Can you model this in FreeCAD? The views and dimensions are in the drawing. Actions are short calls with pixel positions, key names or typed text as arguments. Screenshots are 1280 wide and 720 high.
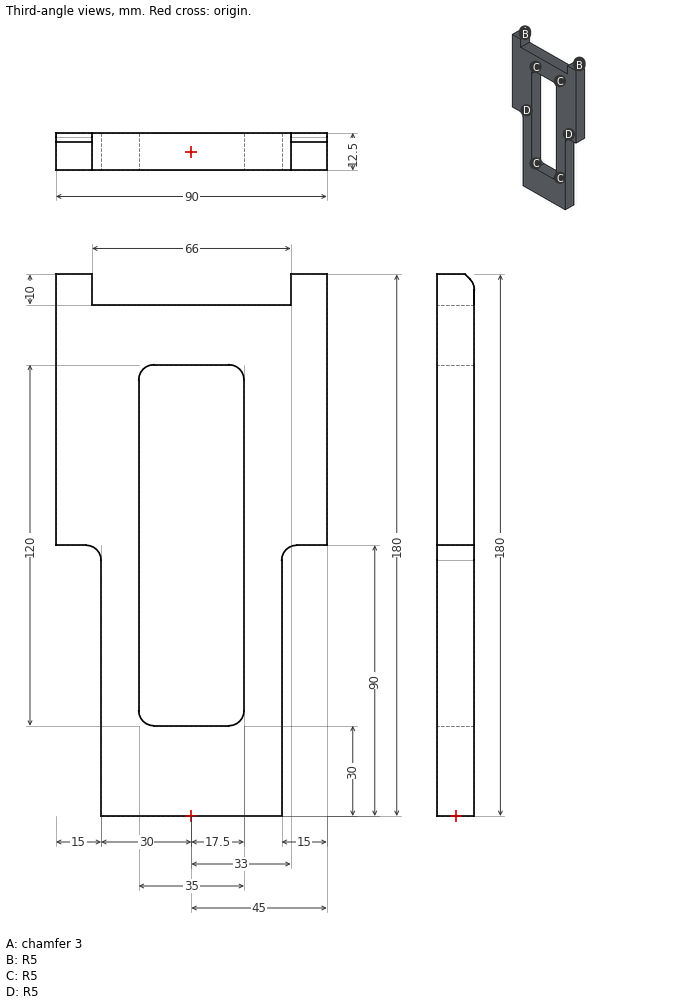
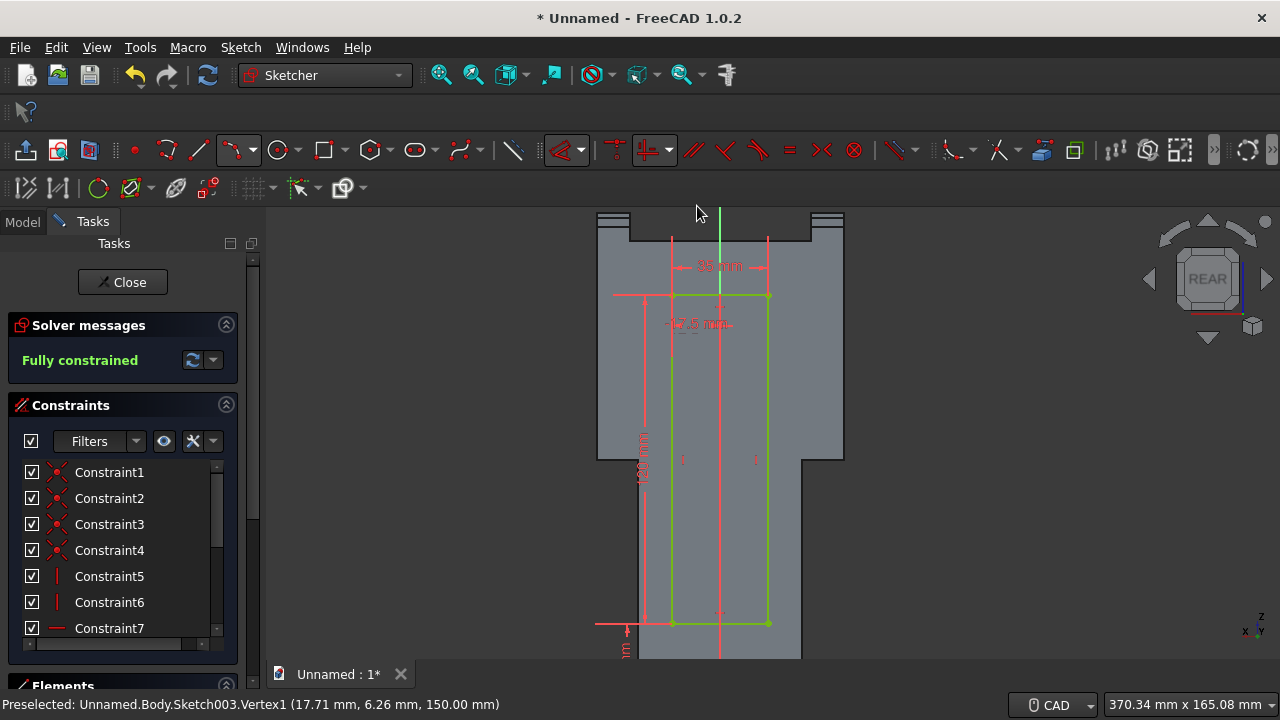
click(123, 282)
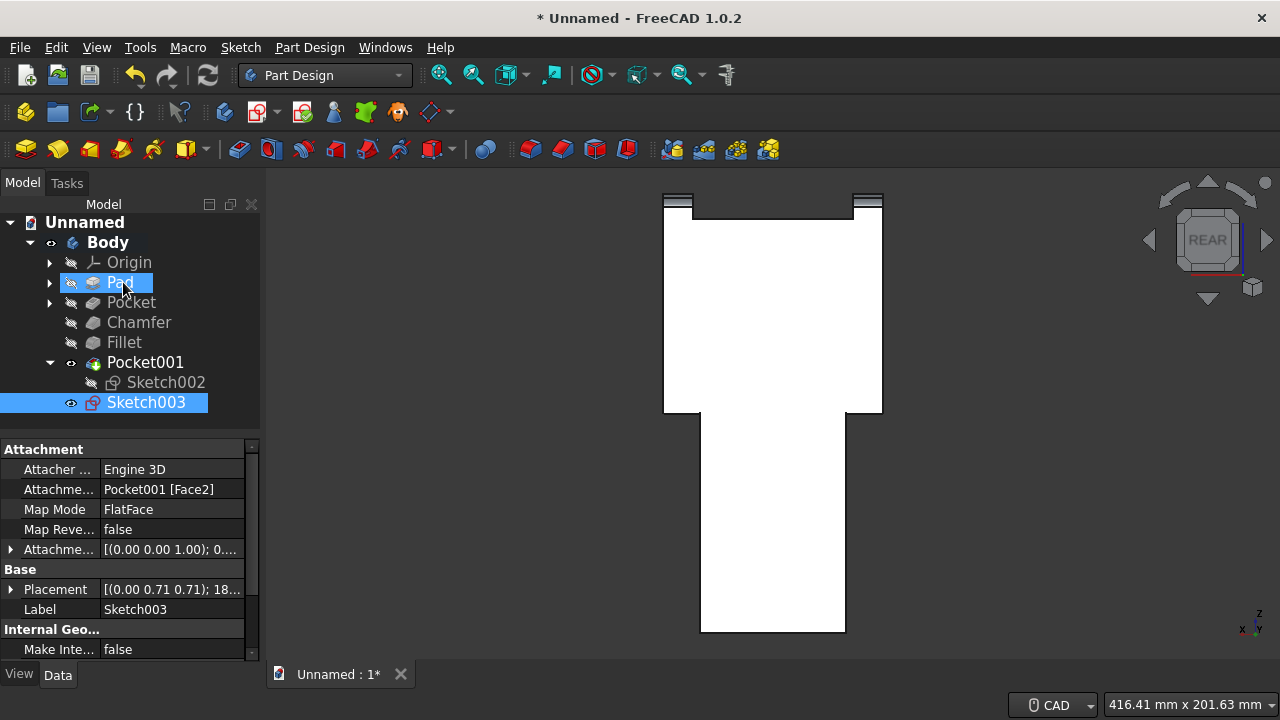
click(240, 150)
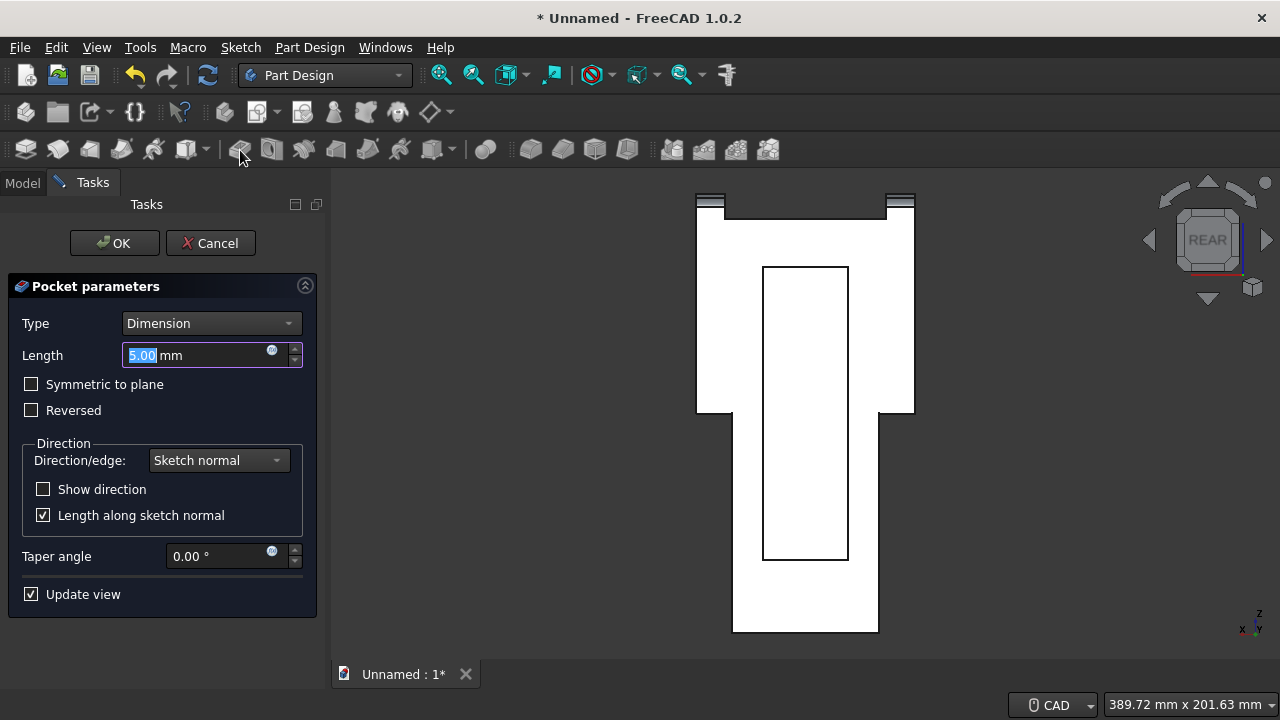
click(212, 324)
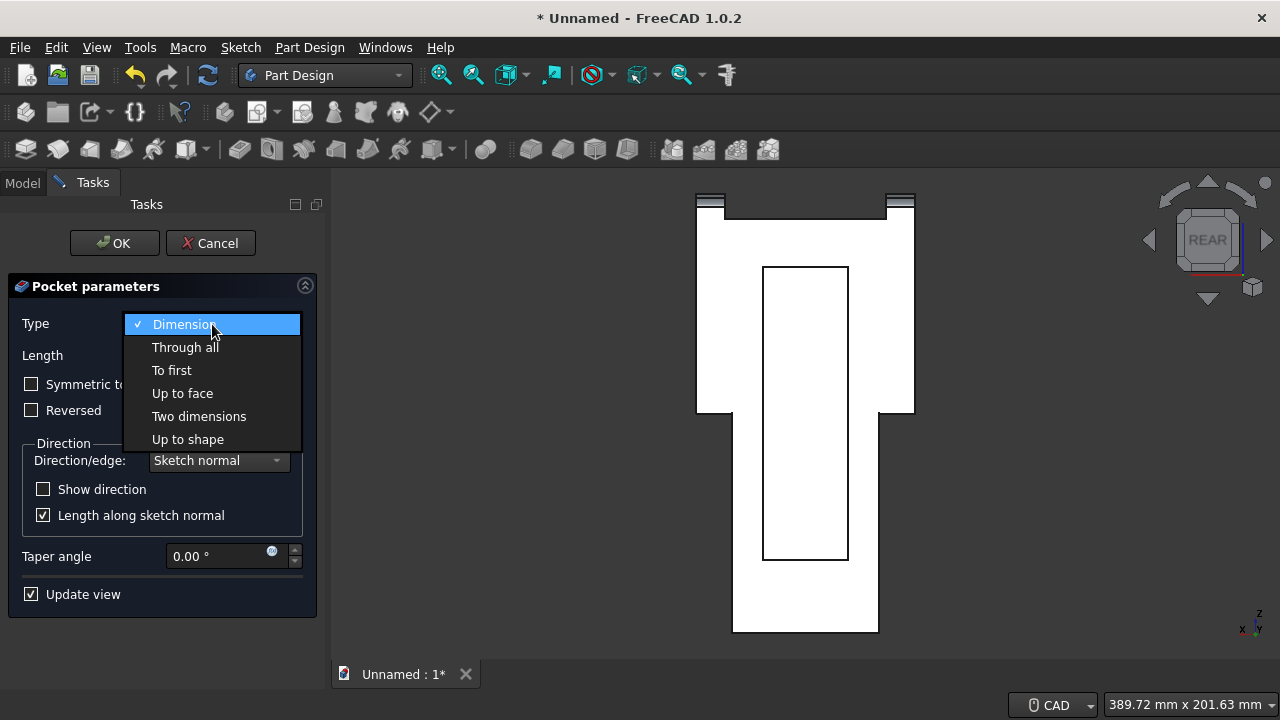
click(212, 348)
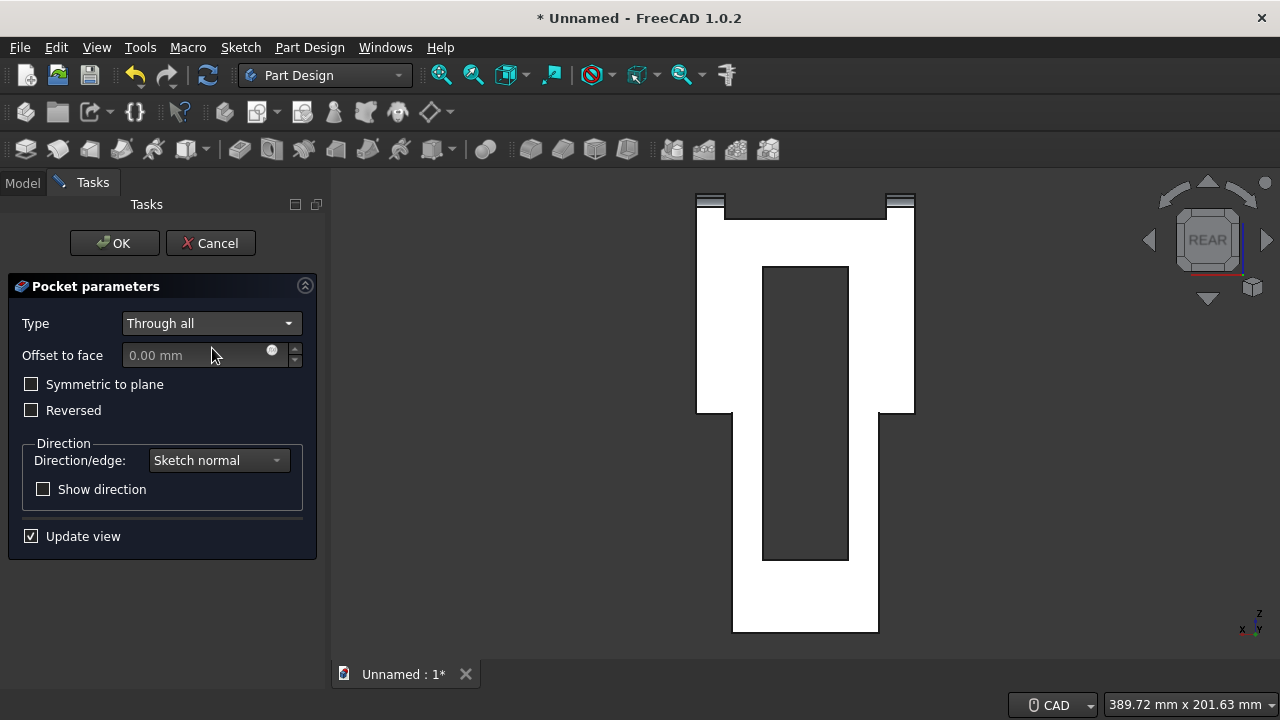
click(115, 243)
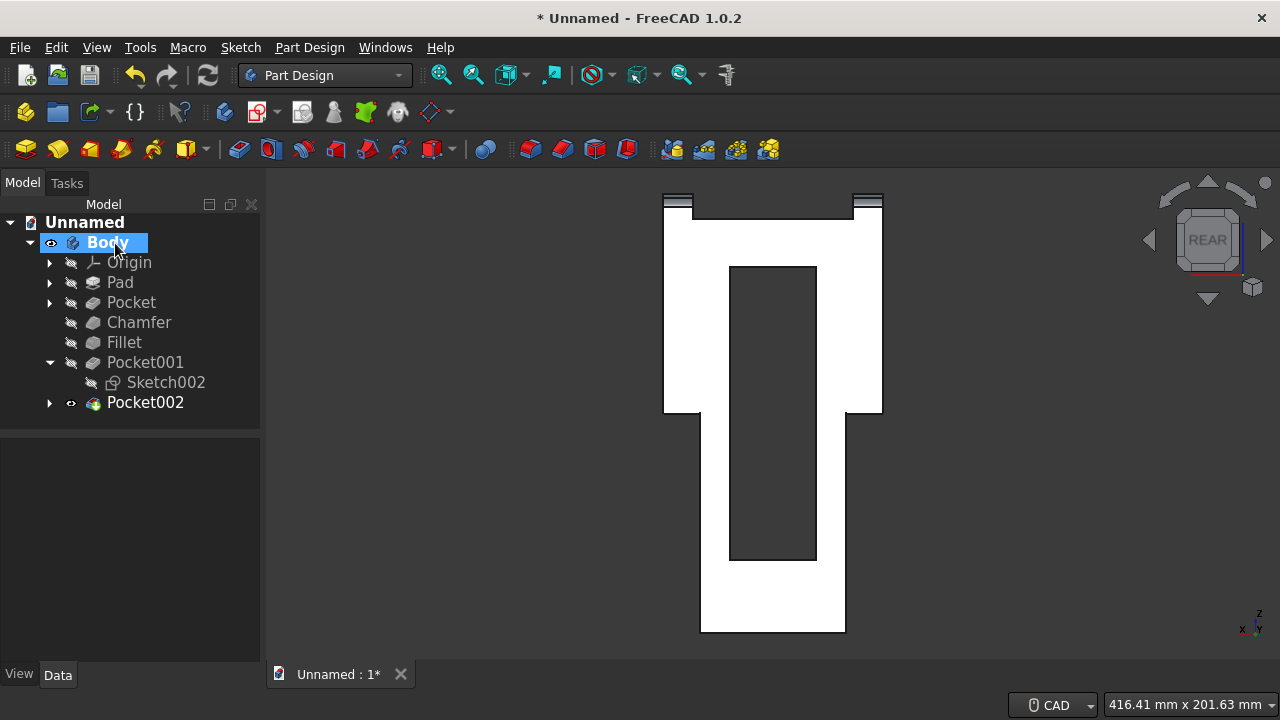
key(0)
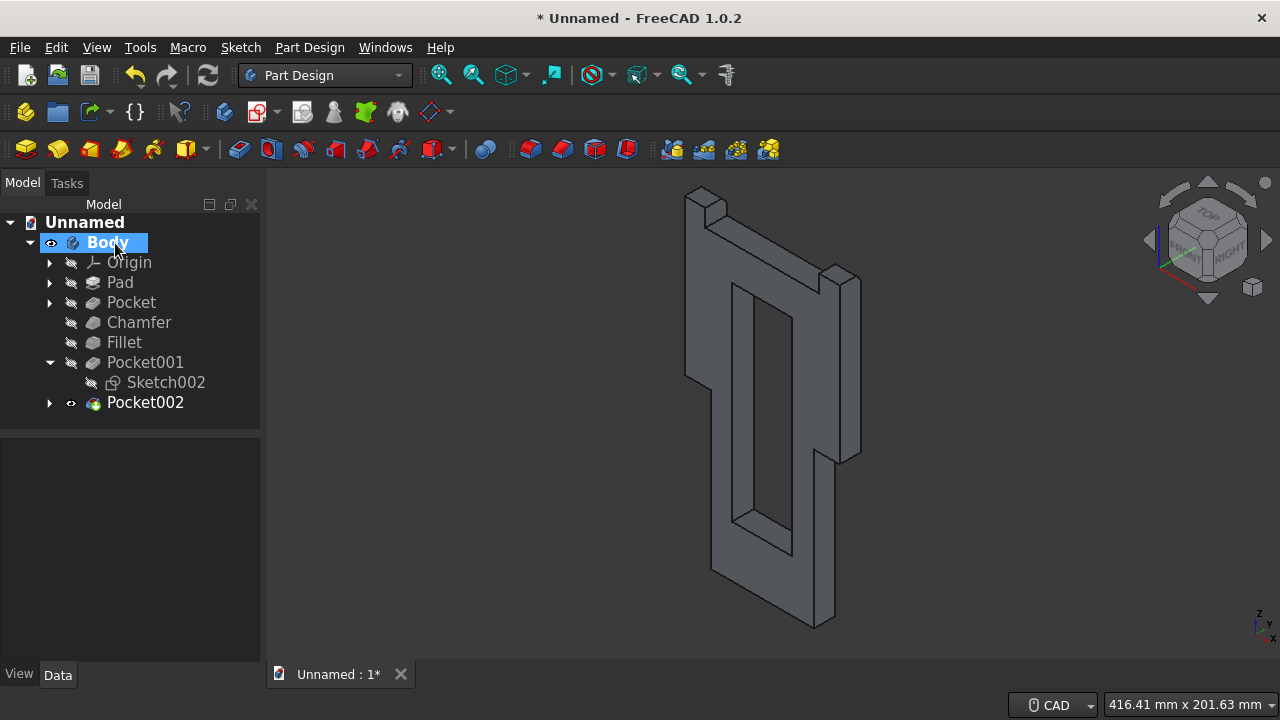
key(2)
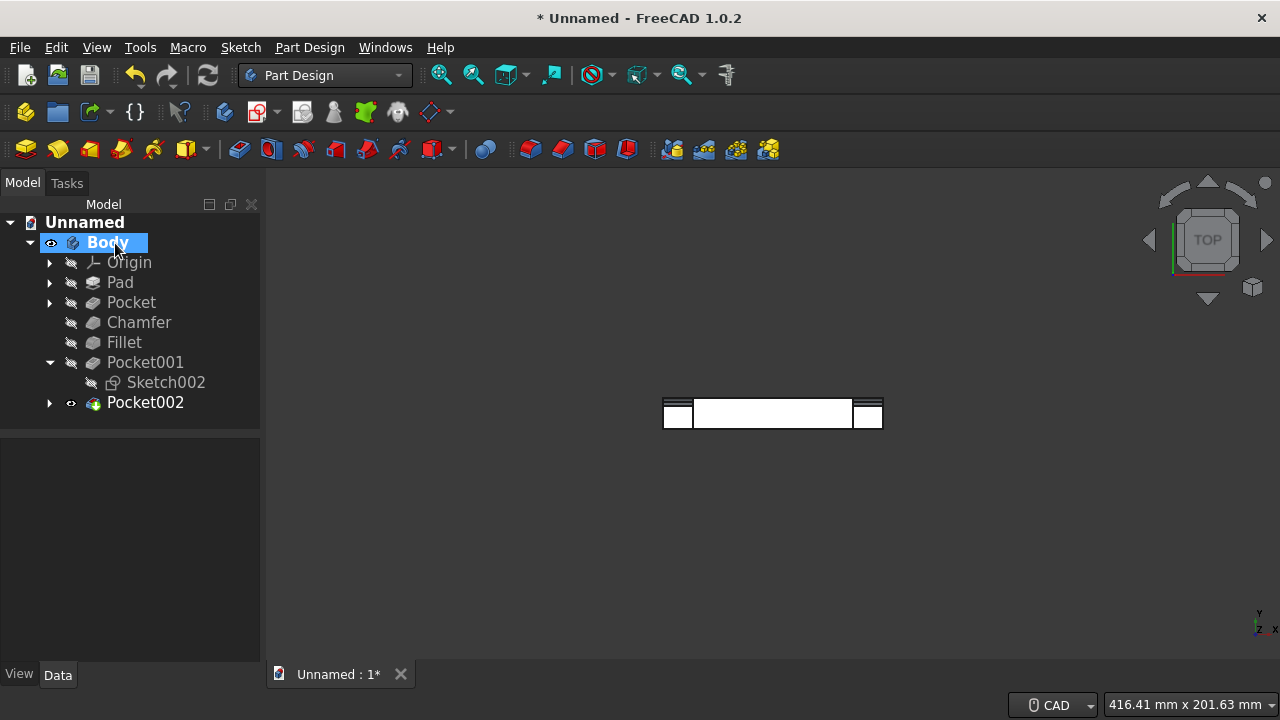
click(442, 76)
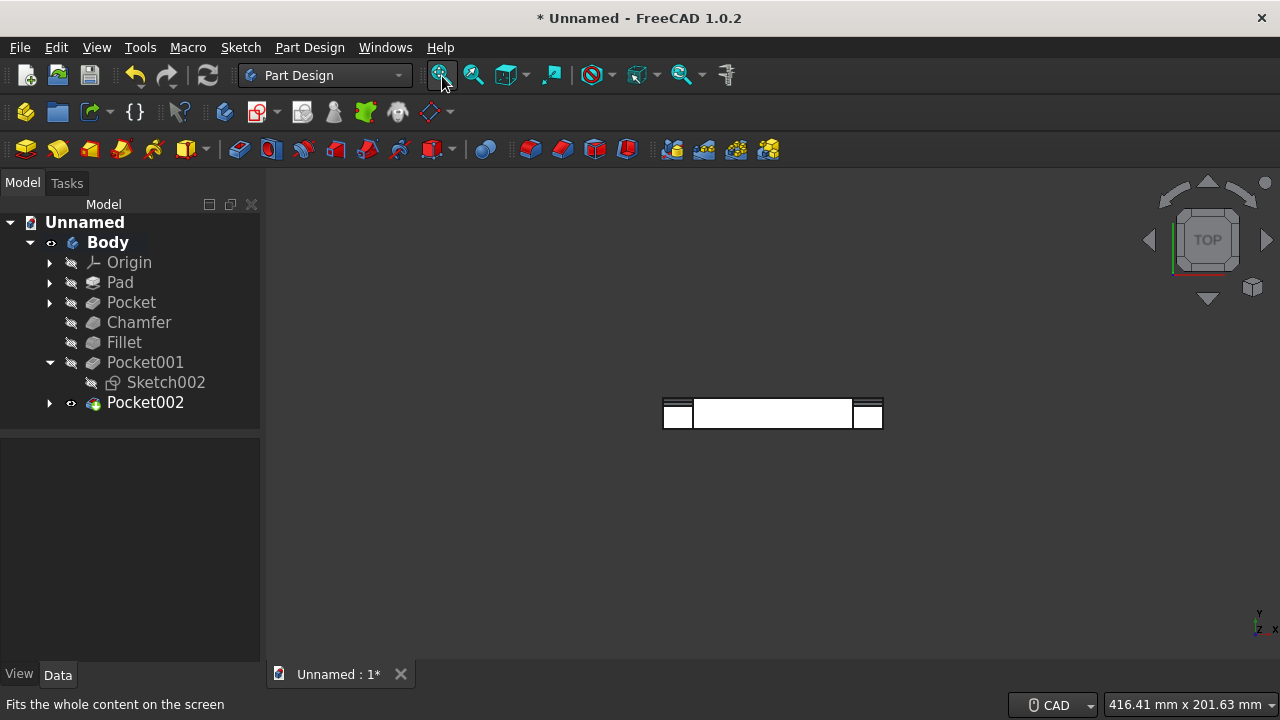
key(1)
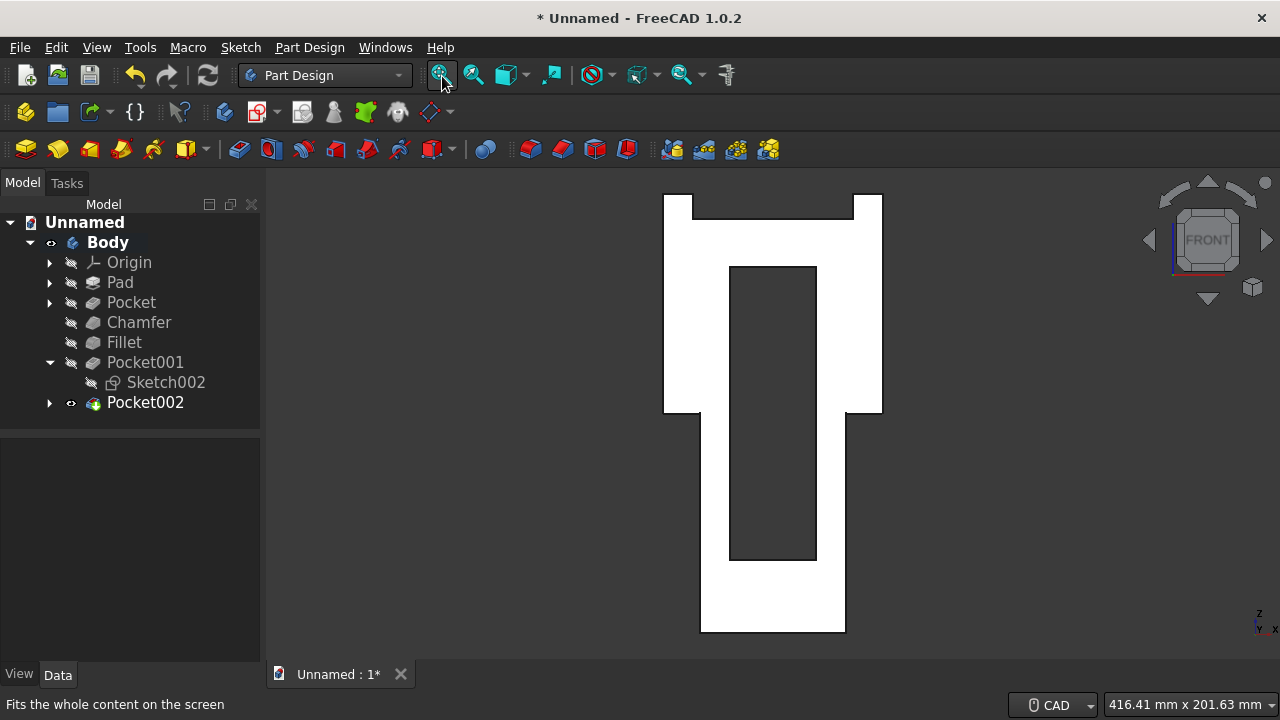
key(3)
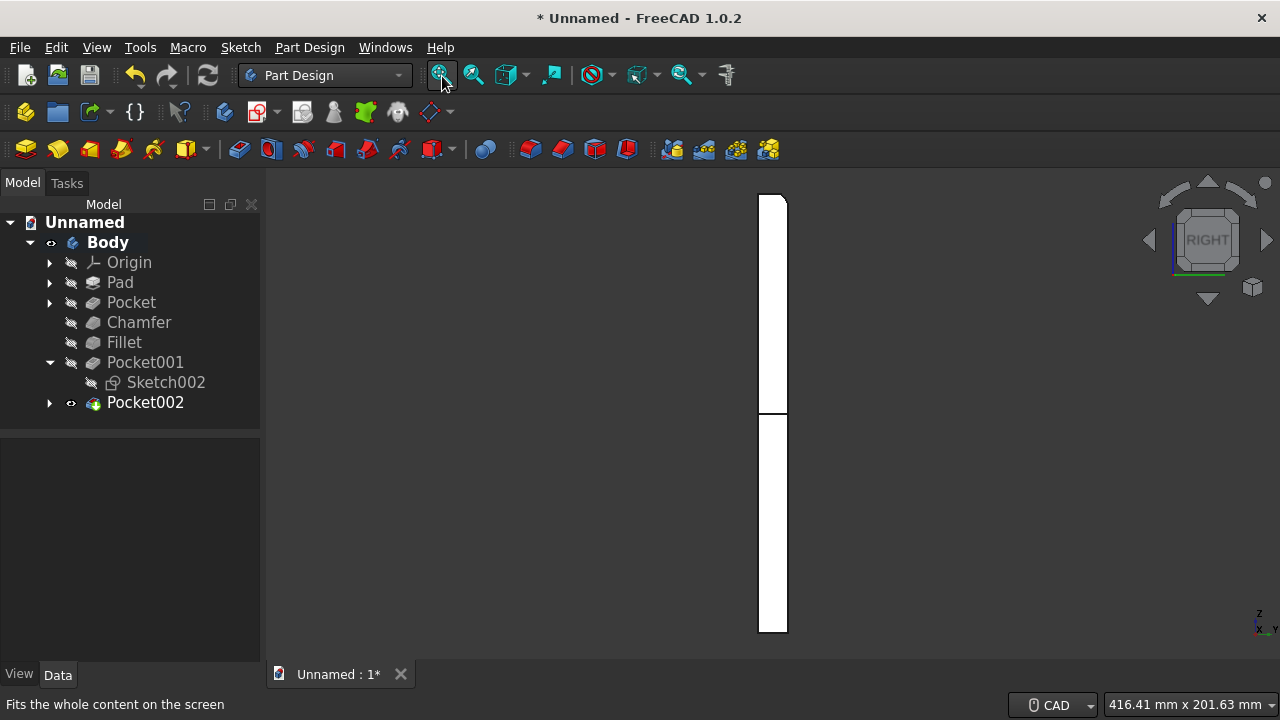
key(5)